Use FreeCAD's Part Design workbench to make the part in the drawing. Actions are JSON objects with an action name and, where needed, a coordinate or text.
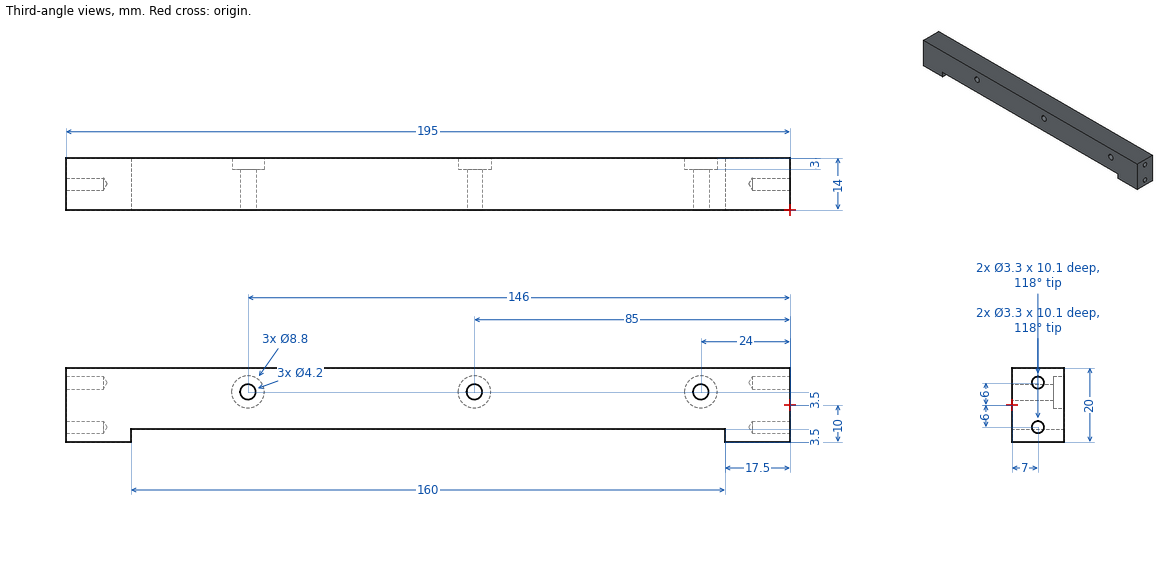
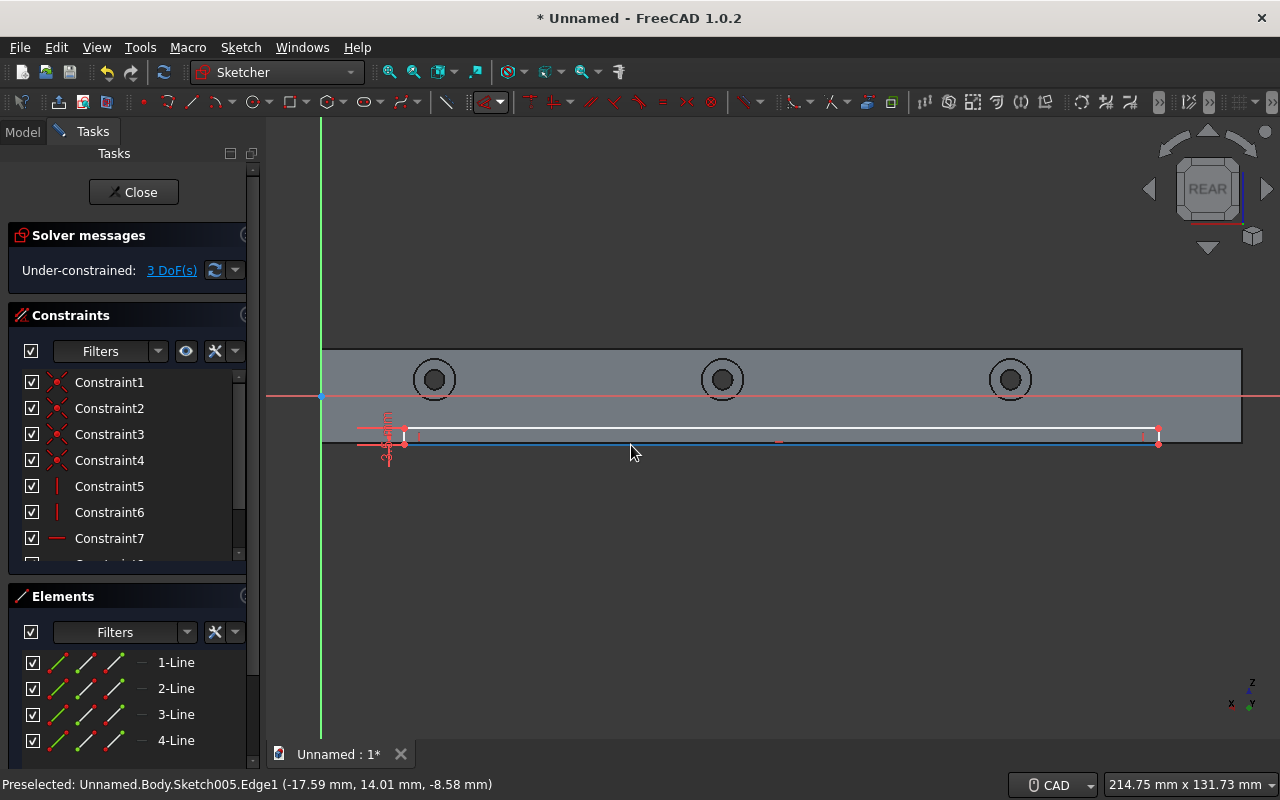
{"action": "left_click", "coordinate": [631, 445]}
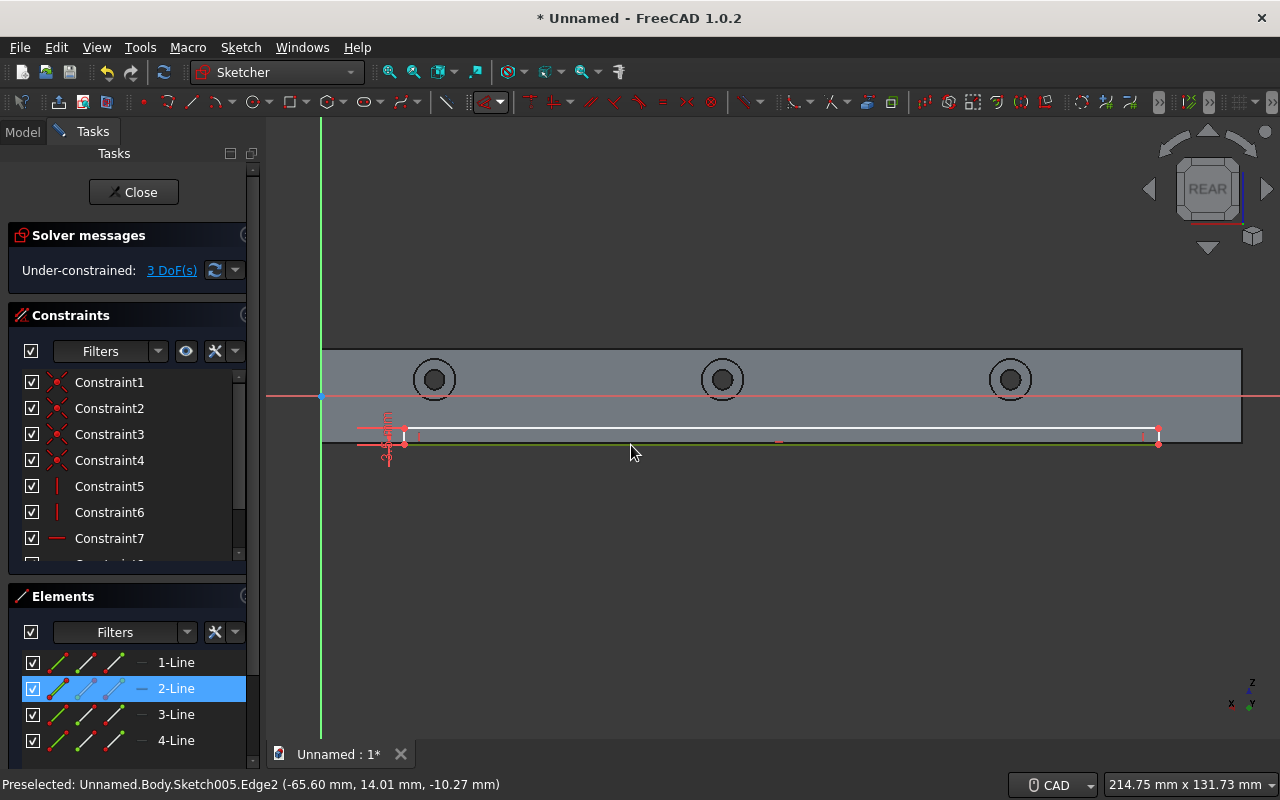
{"action": "key", "text": "l"}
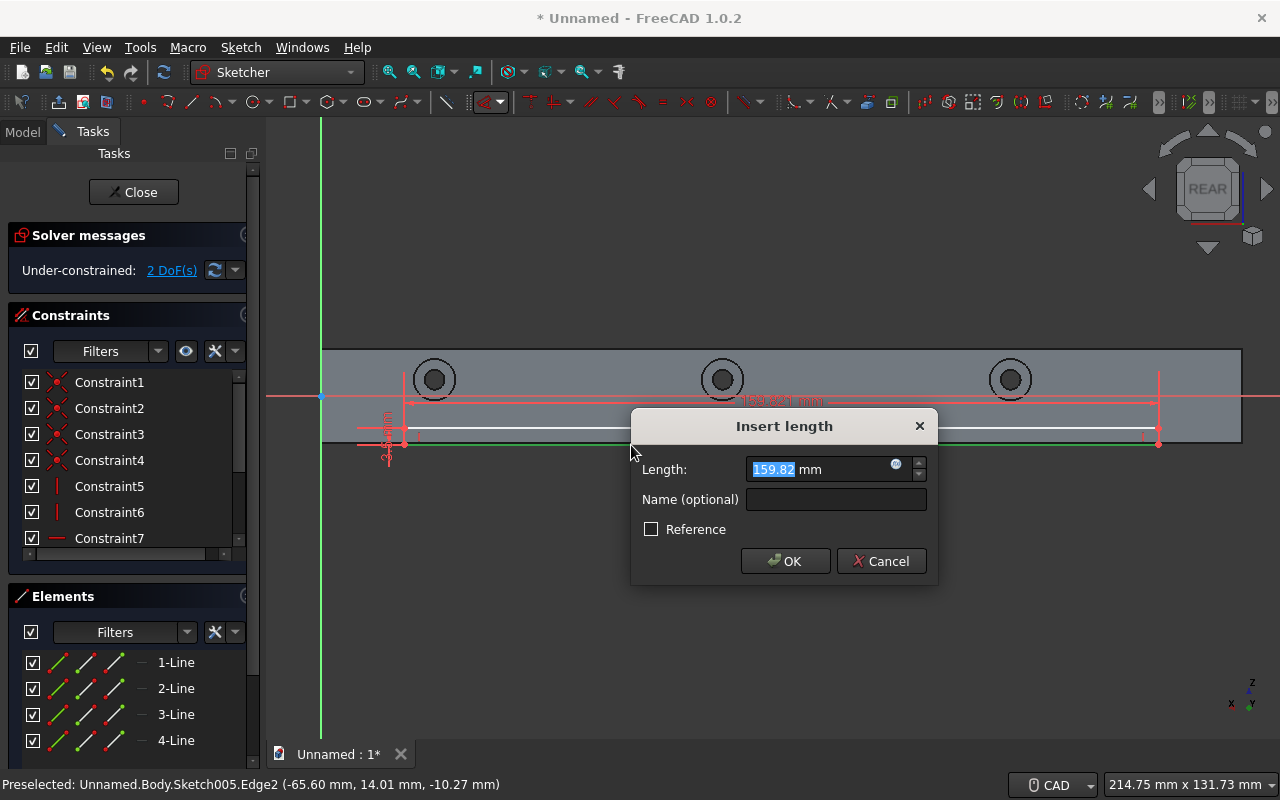
{"action": "type", "text": "160"}
{"action": "key", "text": "Return"}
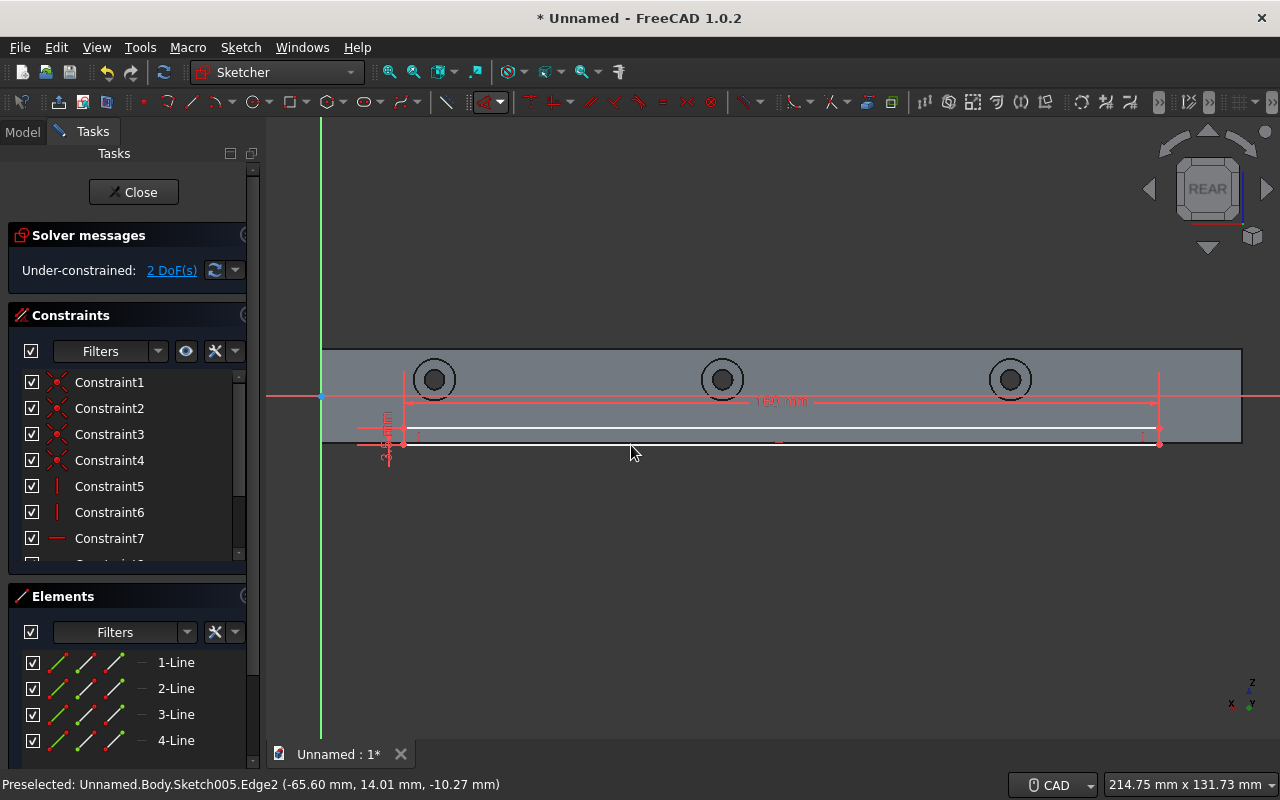
{"action": "left_click", "coordinate": [404, 445]}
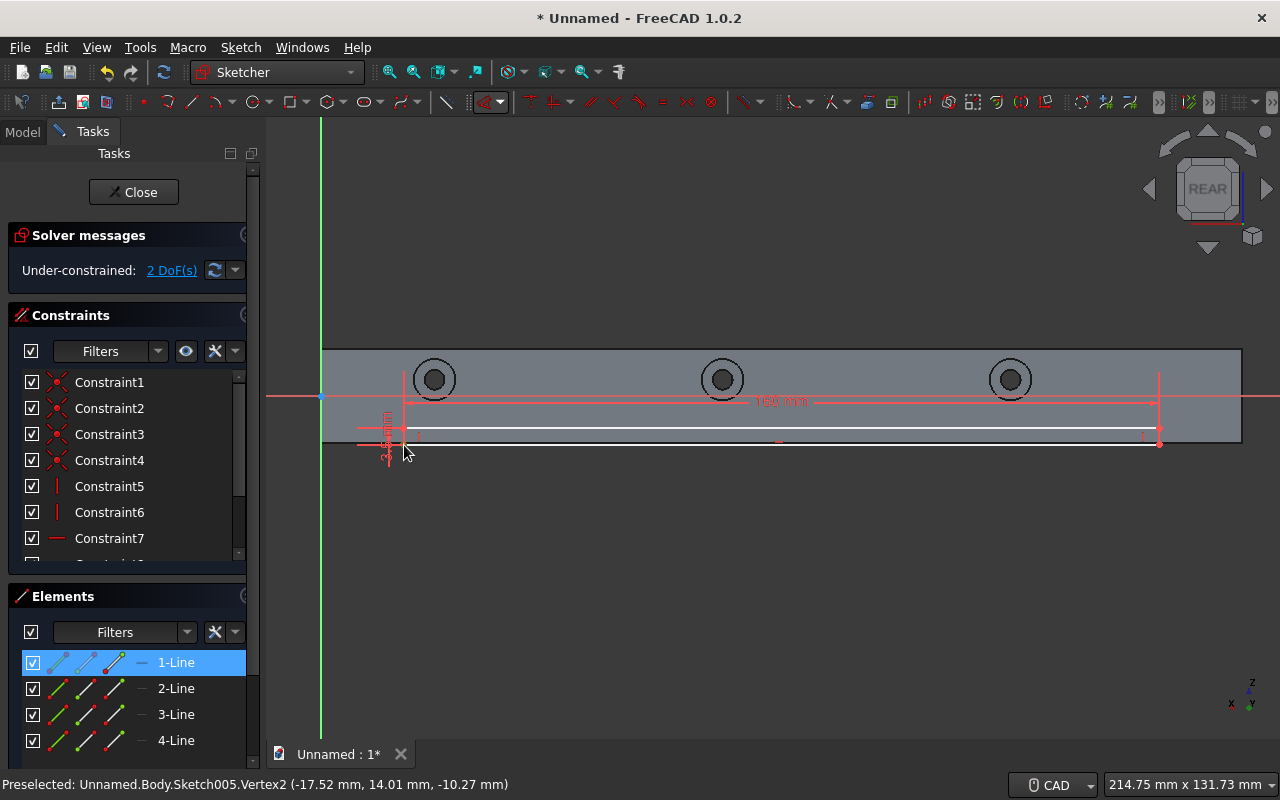
{"action": "key", "text": "i"}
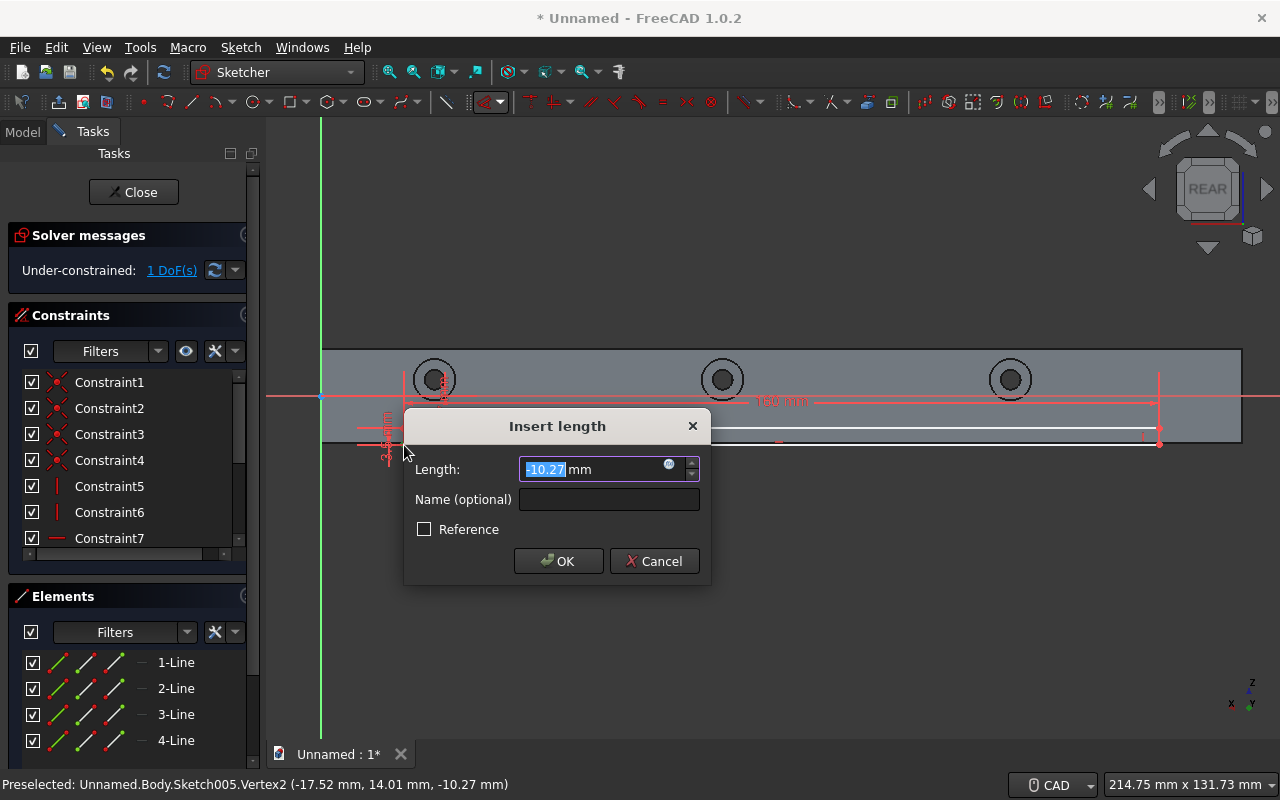
{"action": "type", "text": "-10"}
{"action": "key", "text": "Return"}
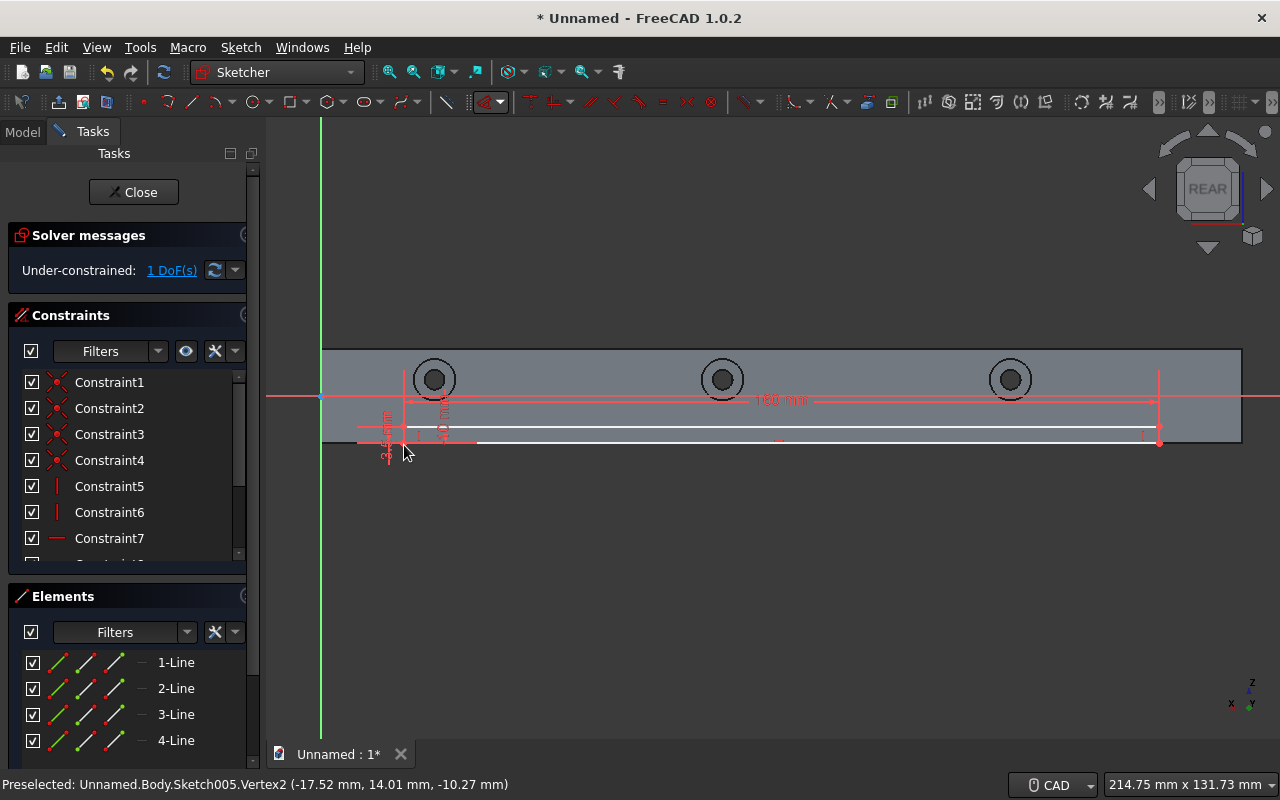
{"action": "left_click", "coordinate": [404, 427]}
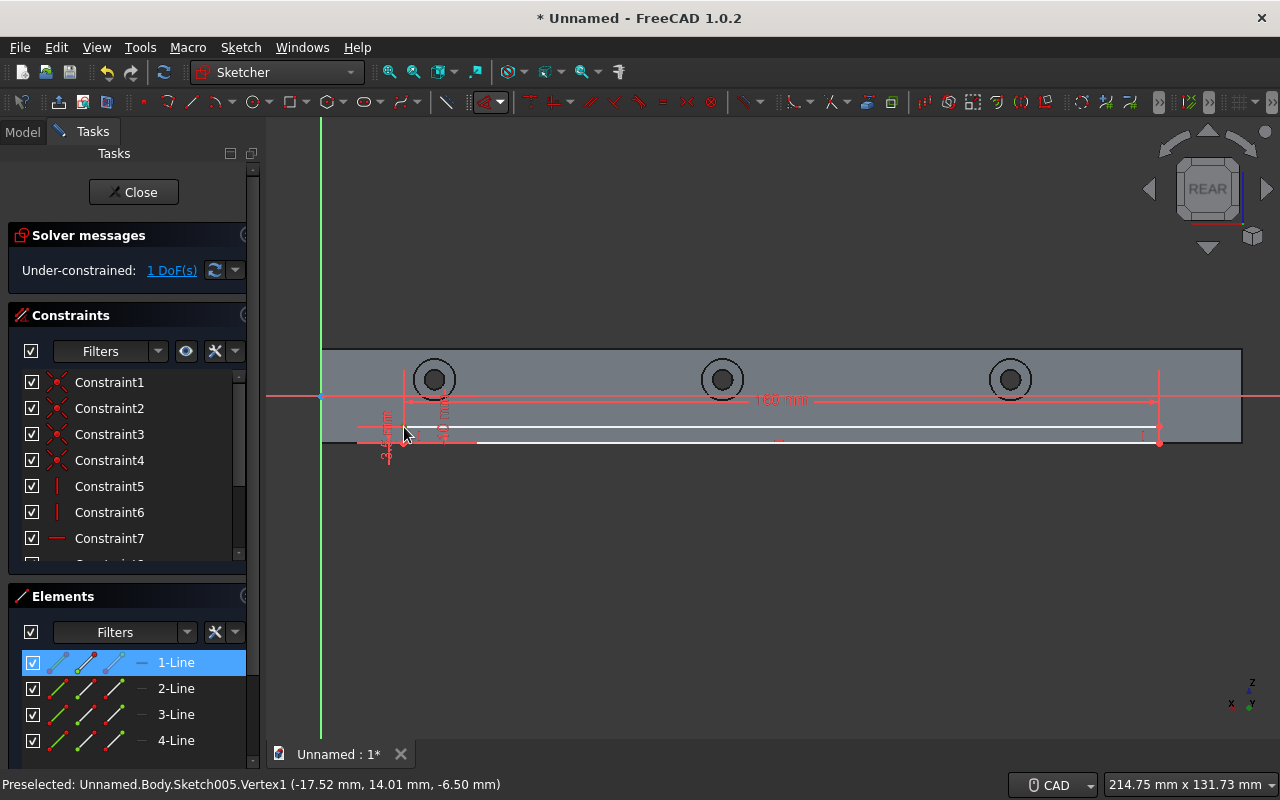
{"action": "key", "text": "l"}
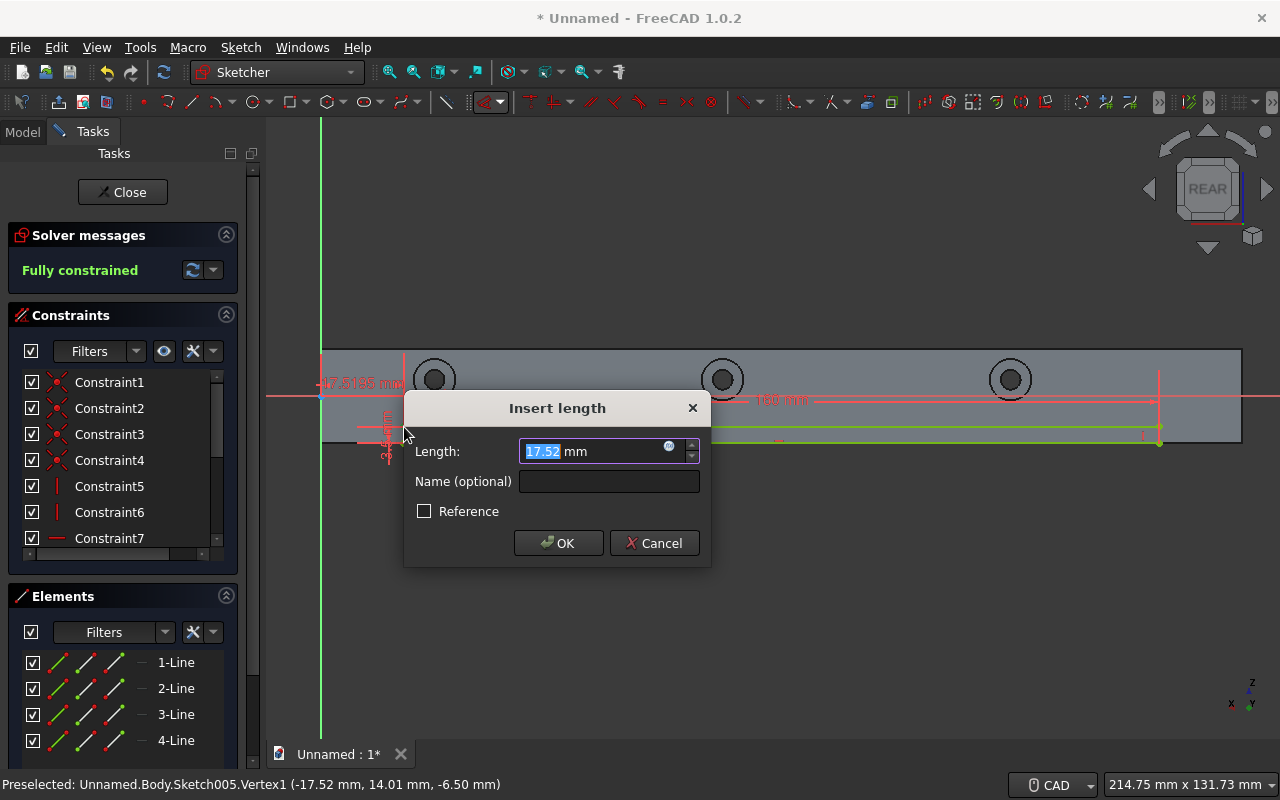
{"action": "type", "text": "17.5"}
{"action": "key", "text": "Return"}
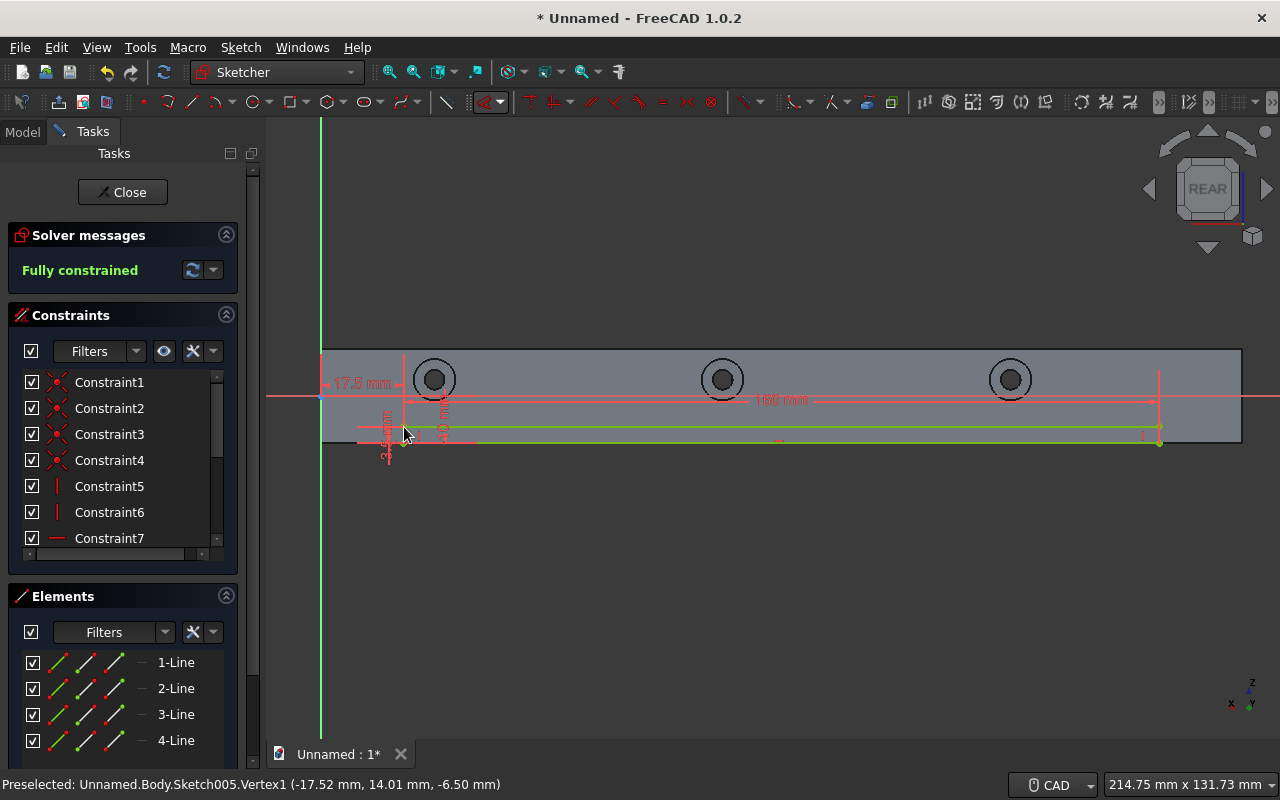
{"action": "left_click", "coordinate": [123, 192]}